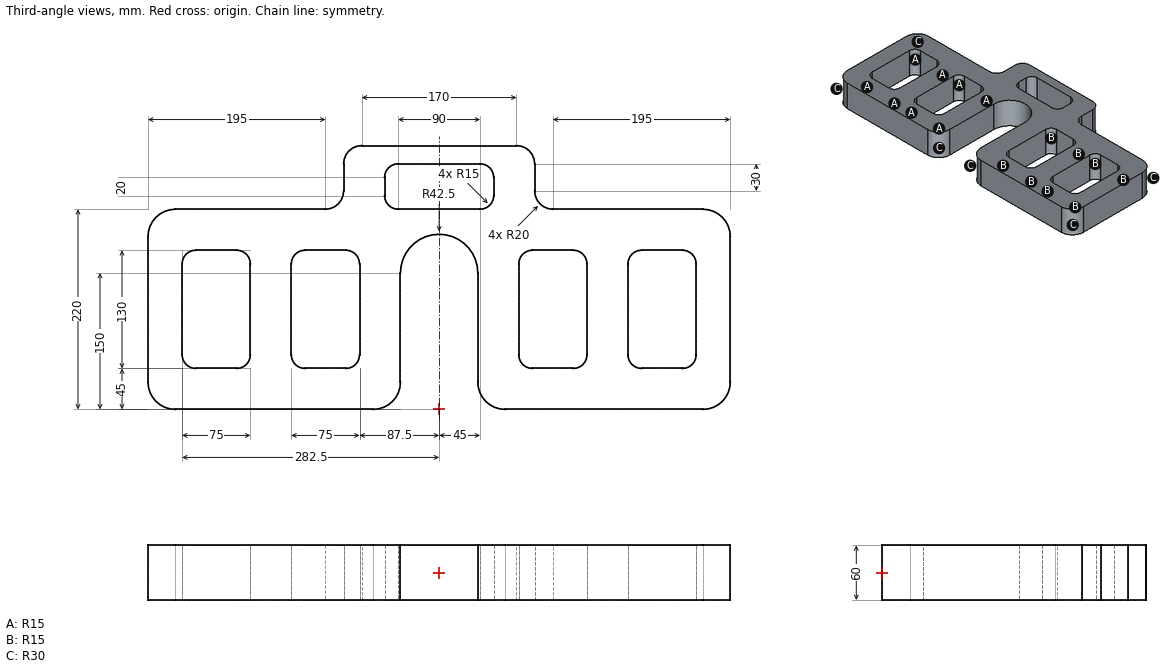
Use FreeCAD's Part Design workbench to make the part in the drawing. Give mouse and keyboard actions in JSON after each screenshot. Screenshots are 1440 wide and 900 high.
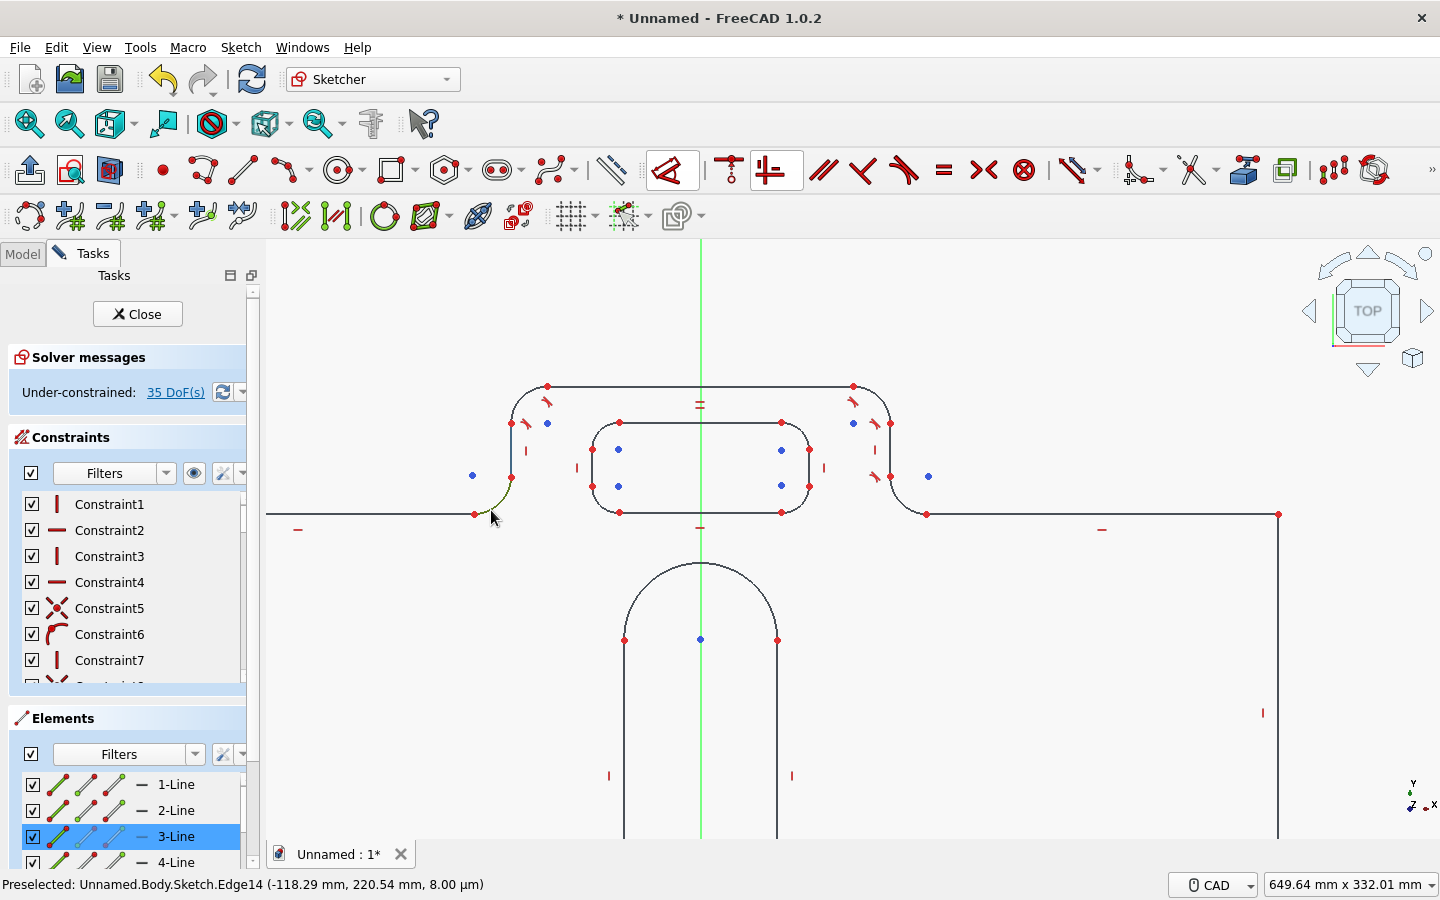
{"action": "left_click", "coordinate": [904, 170]}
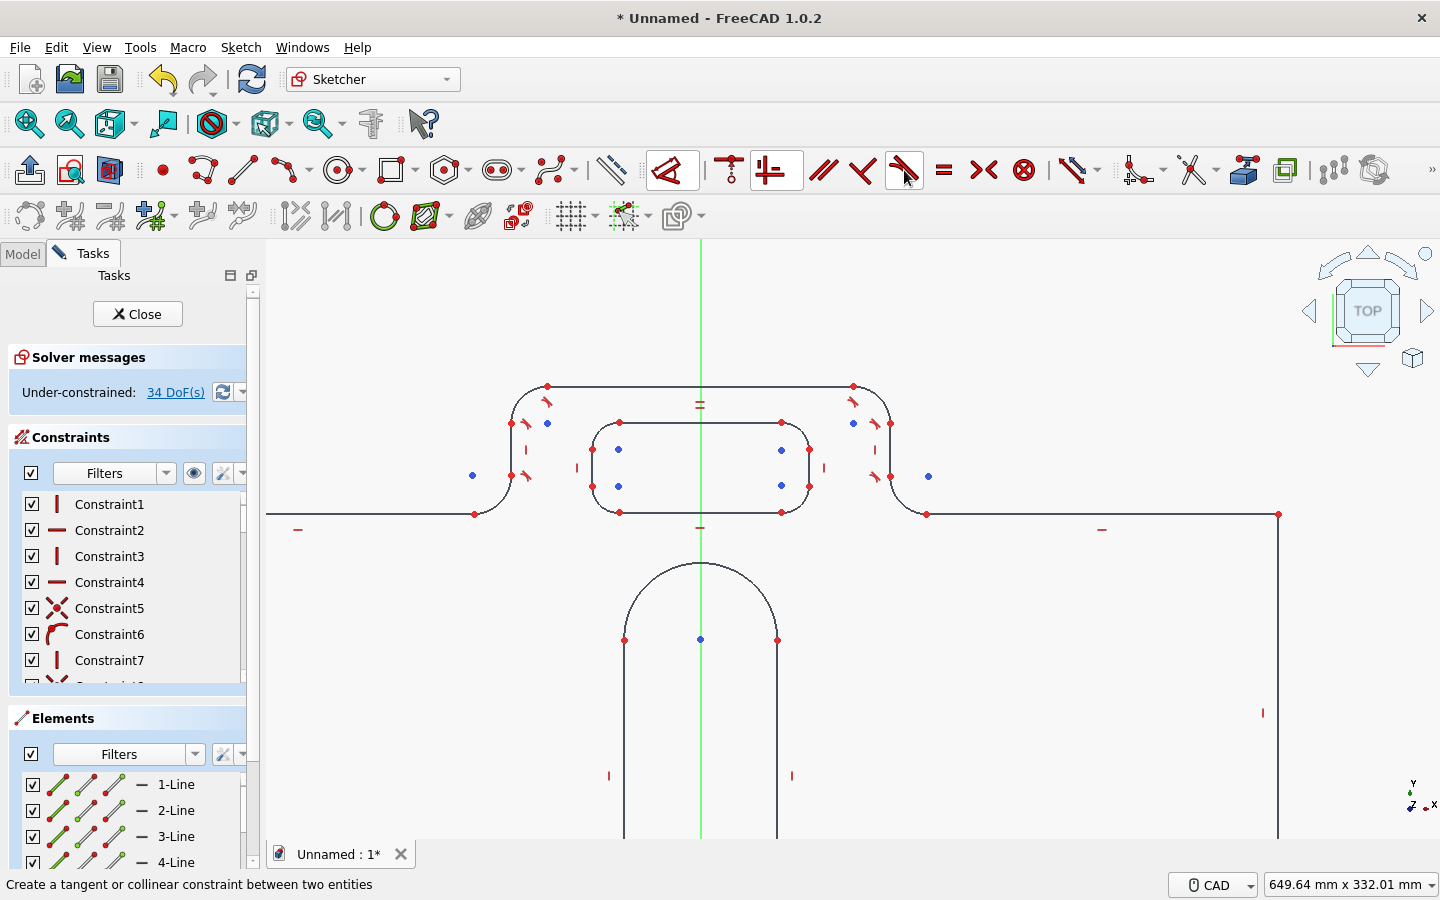
{"action": "left_click", "coordinate": [369, 514]}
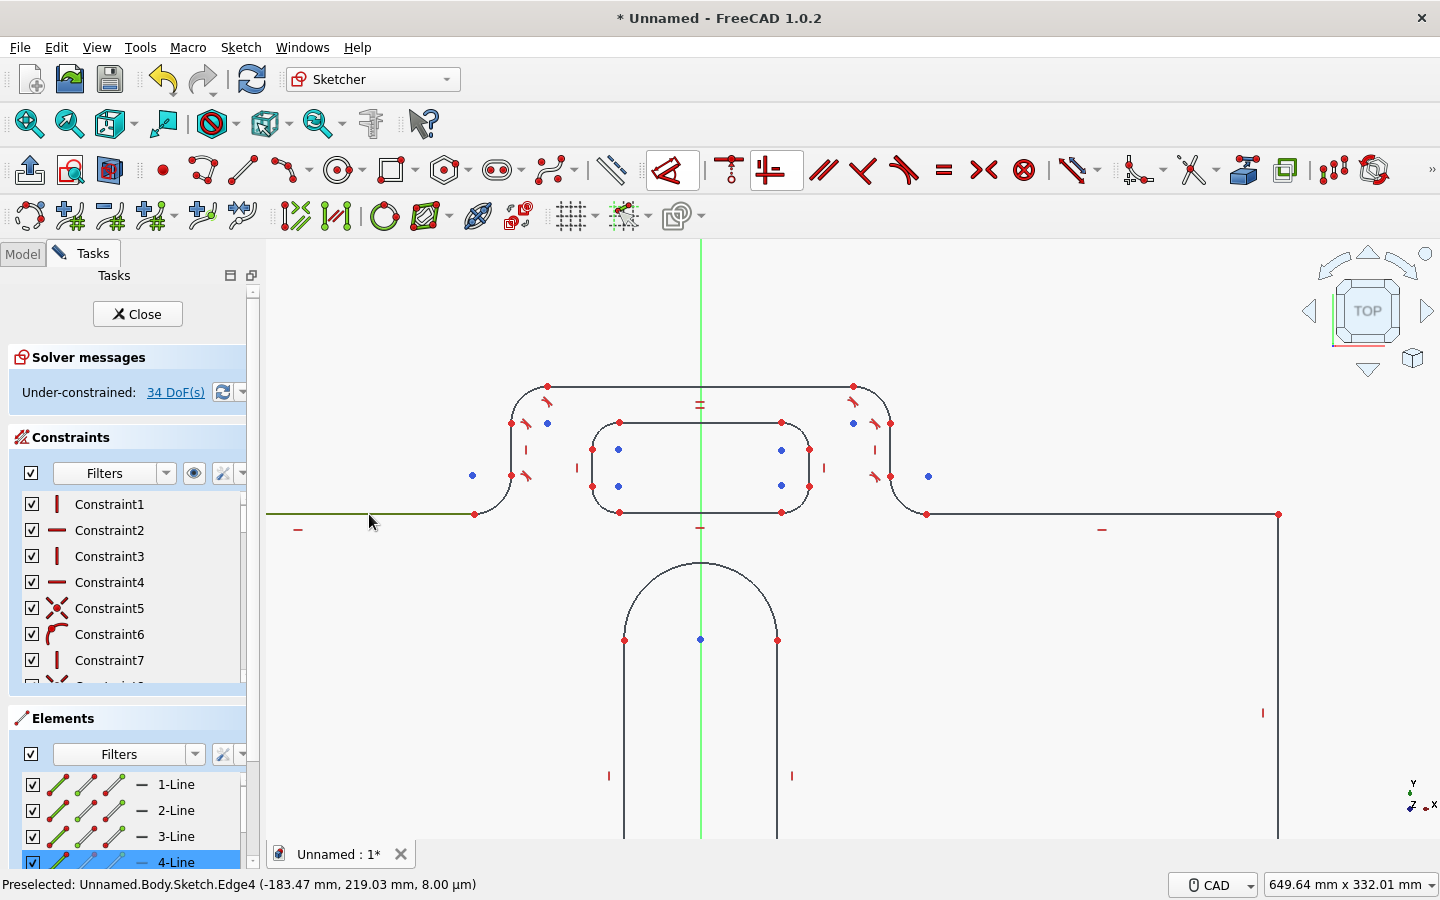
{"action": "left_click", "coordinate": [492, 509]}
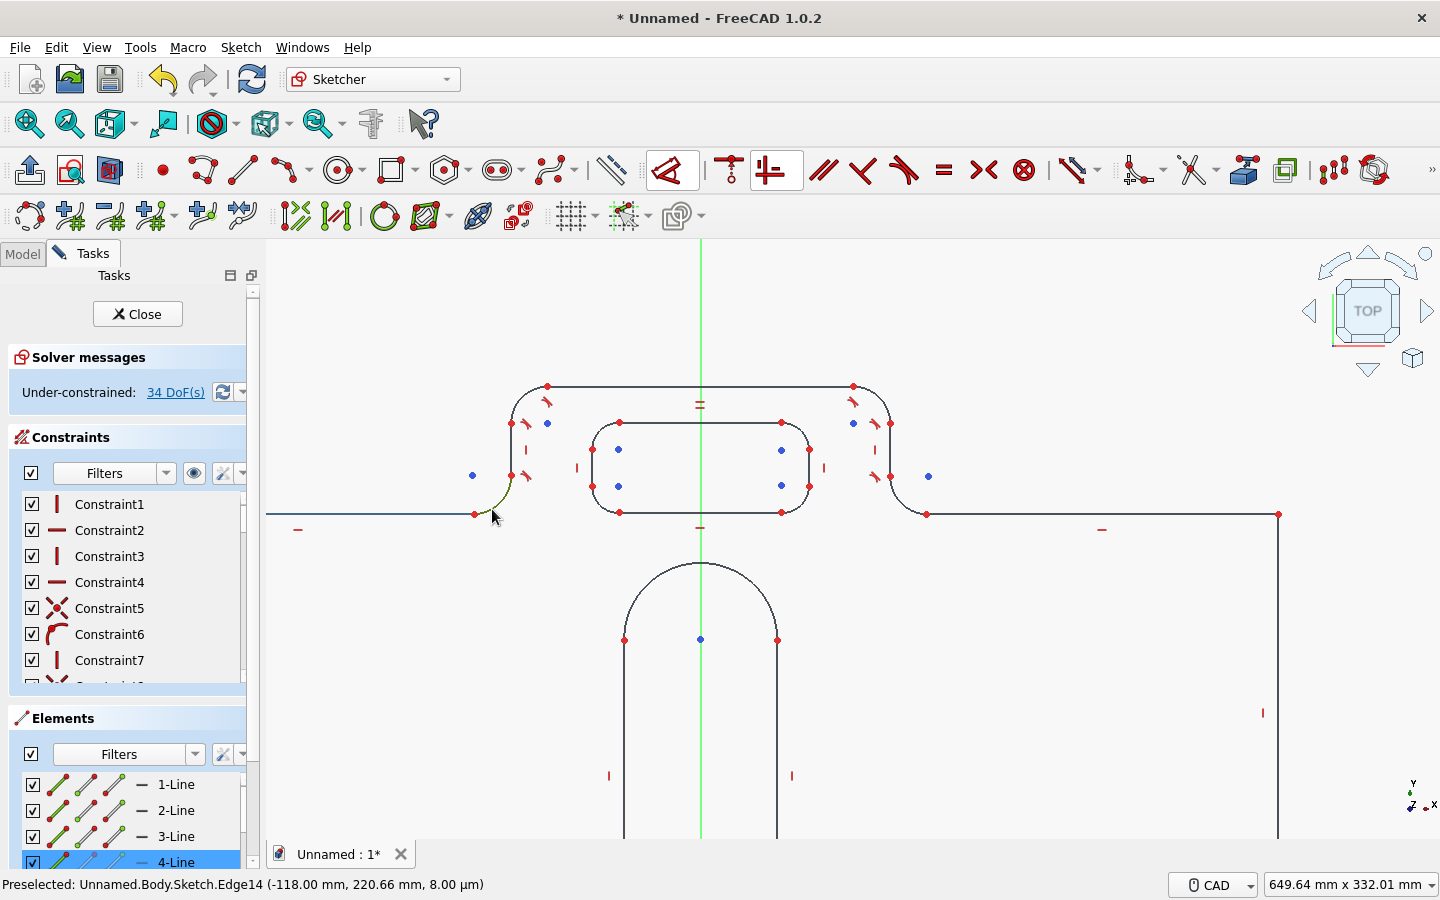
{"action": "left_click", "coordinate": [904, 170]}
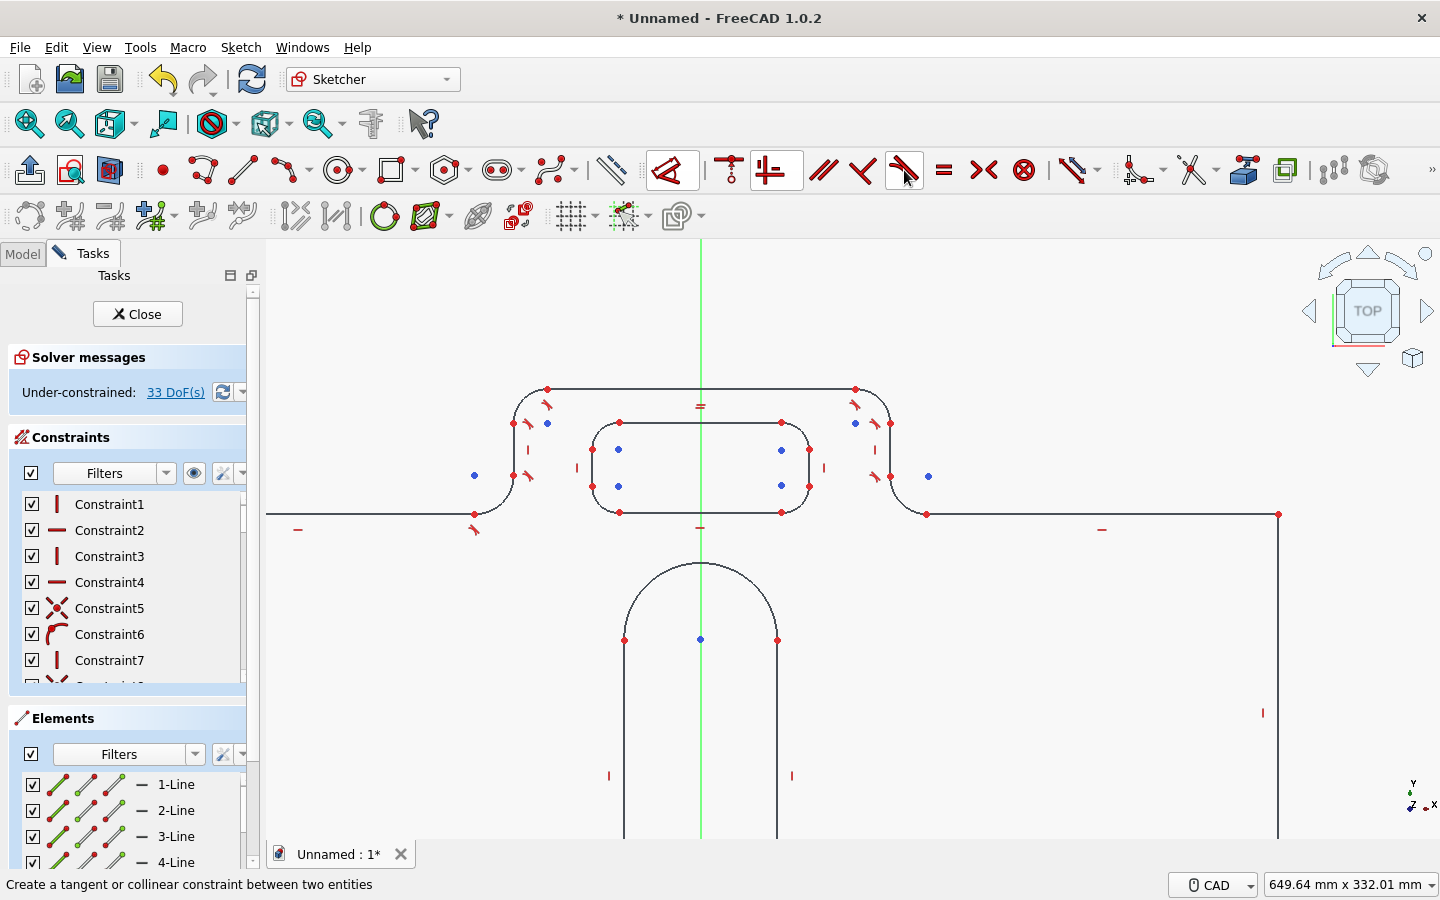
{"action": "left_click", "coordinate": [1173, 514]}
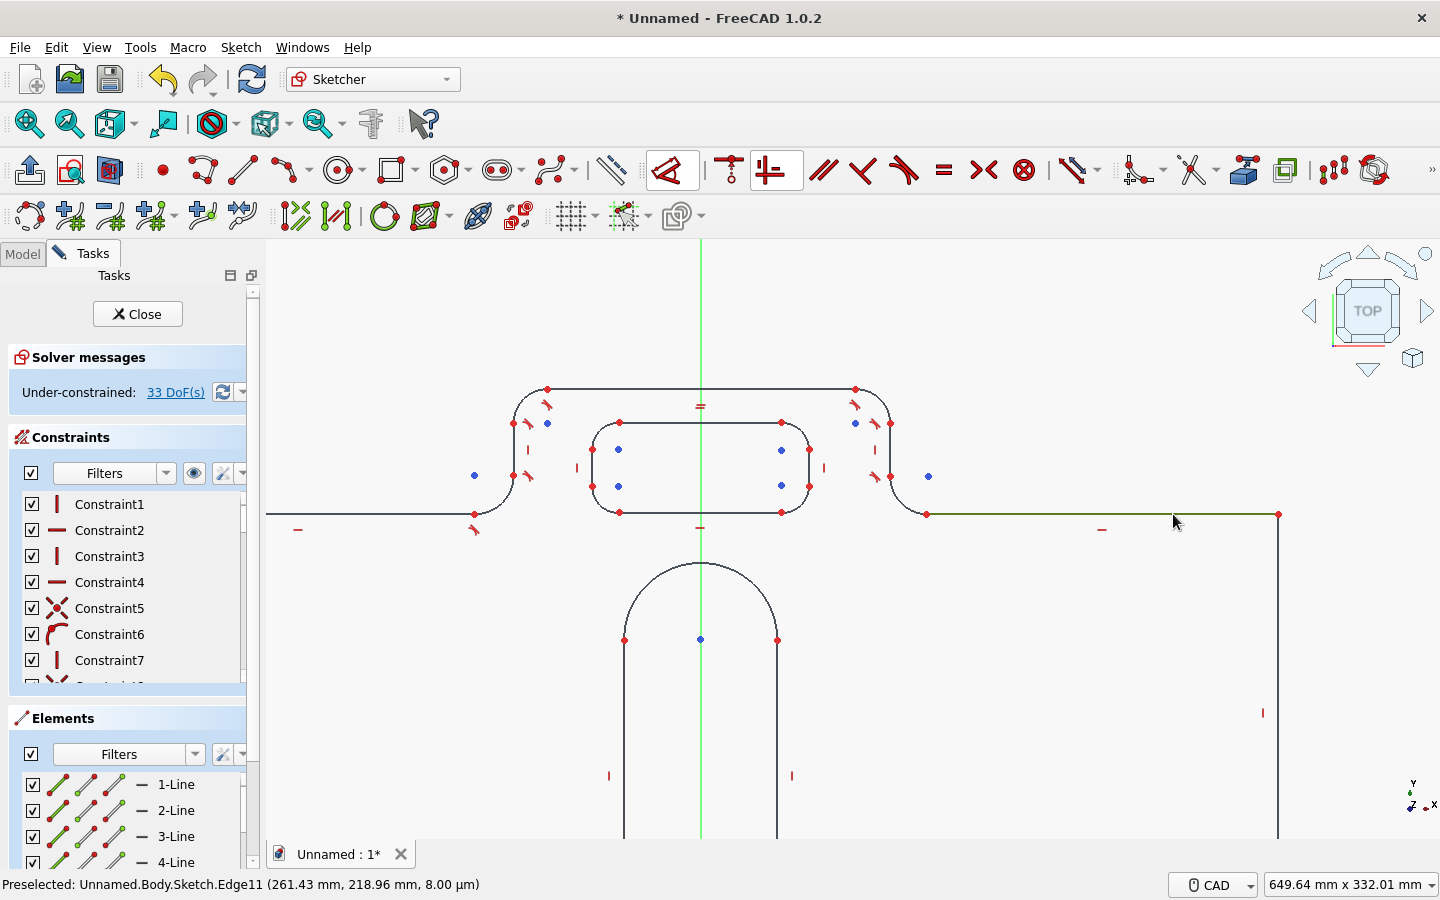
{"action": "left_click", "coordinate": [894, 493]}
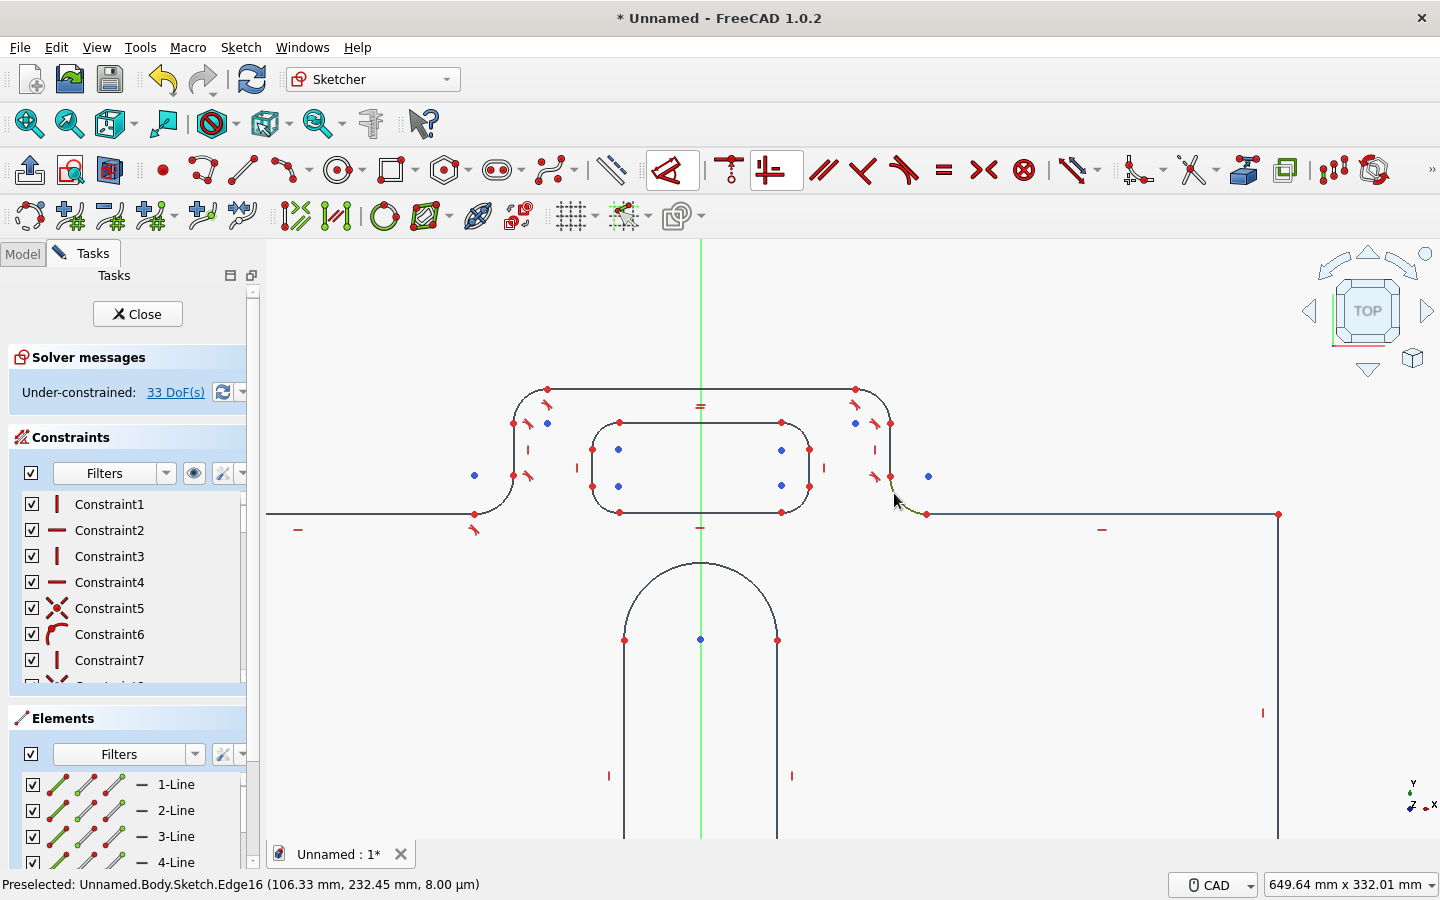
{"action": "left_click", "coordinate": [904, 170]}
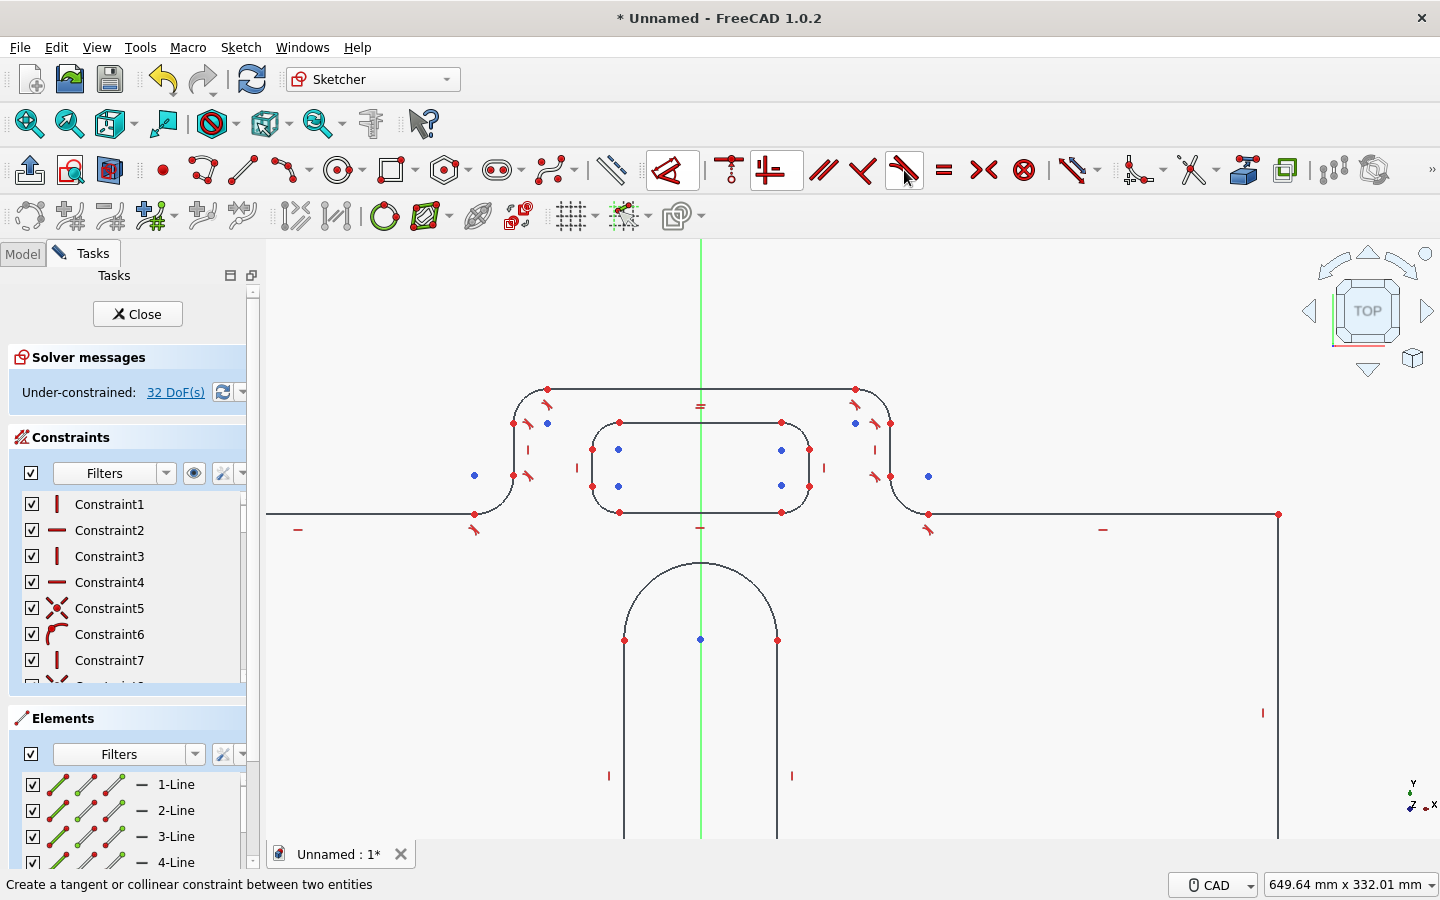
{"action": "left_click", "coordinate": [733, 513]}